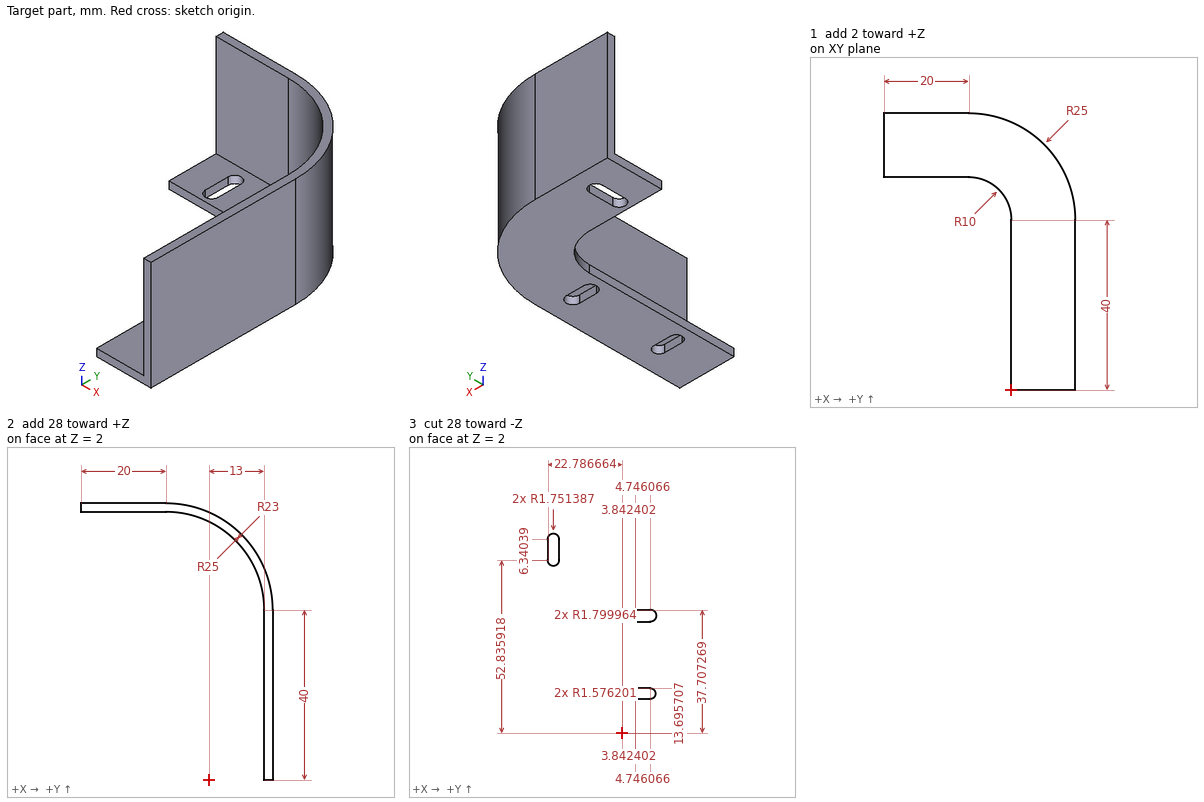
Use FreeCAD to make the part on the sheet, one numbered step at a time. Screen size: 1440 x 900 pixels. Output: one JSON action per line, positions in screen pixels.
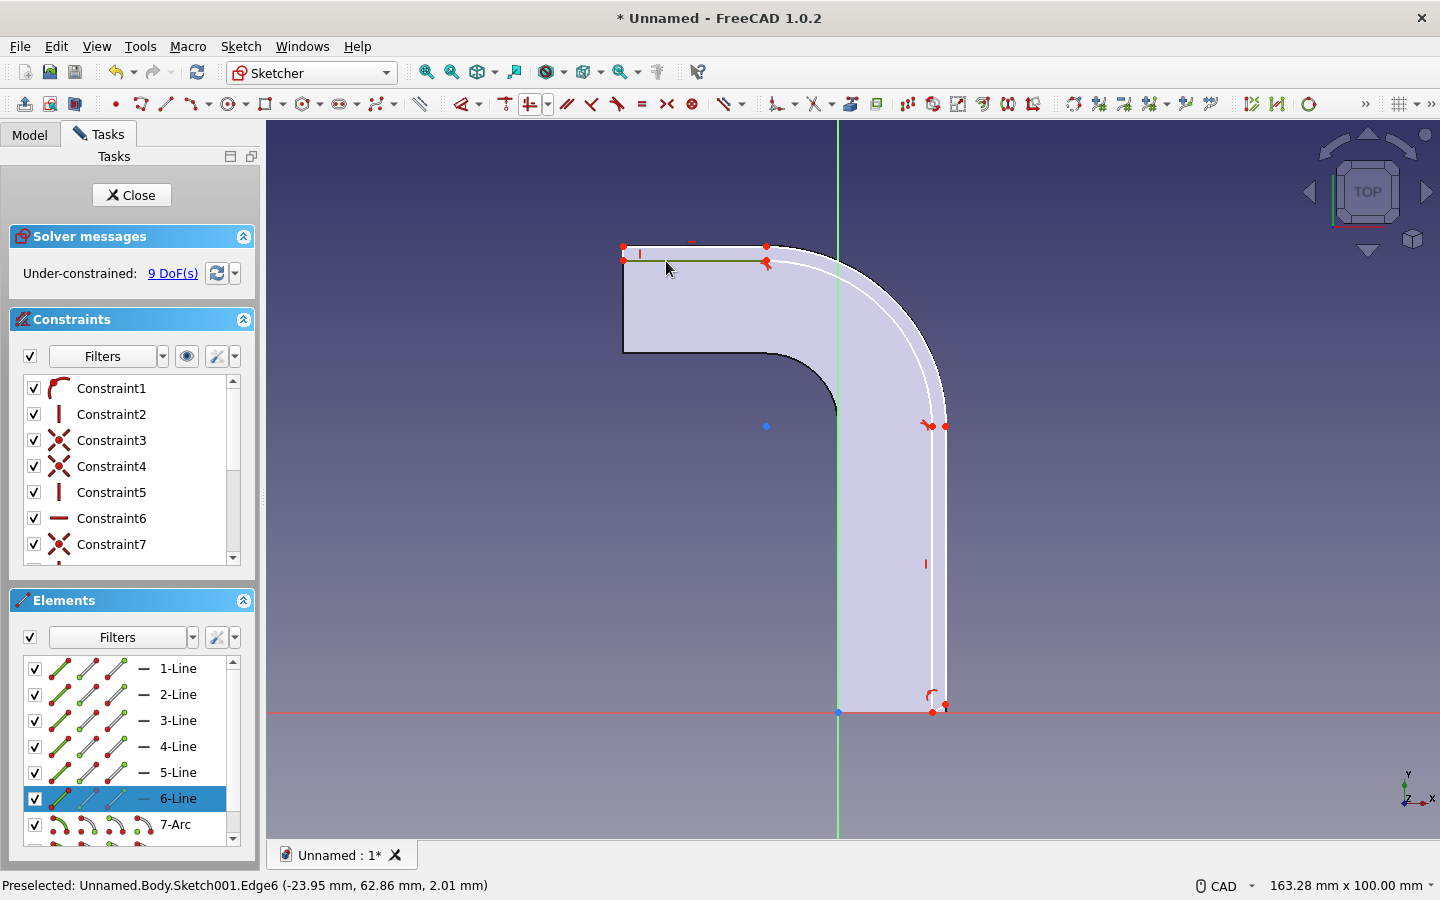
{"action": "left_click", "coordinate": [914, 351]}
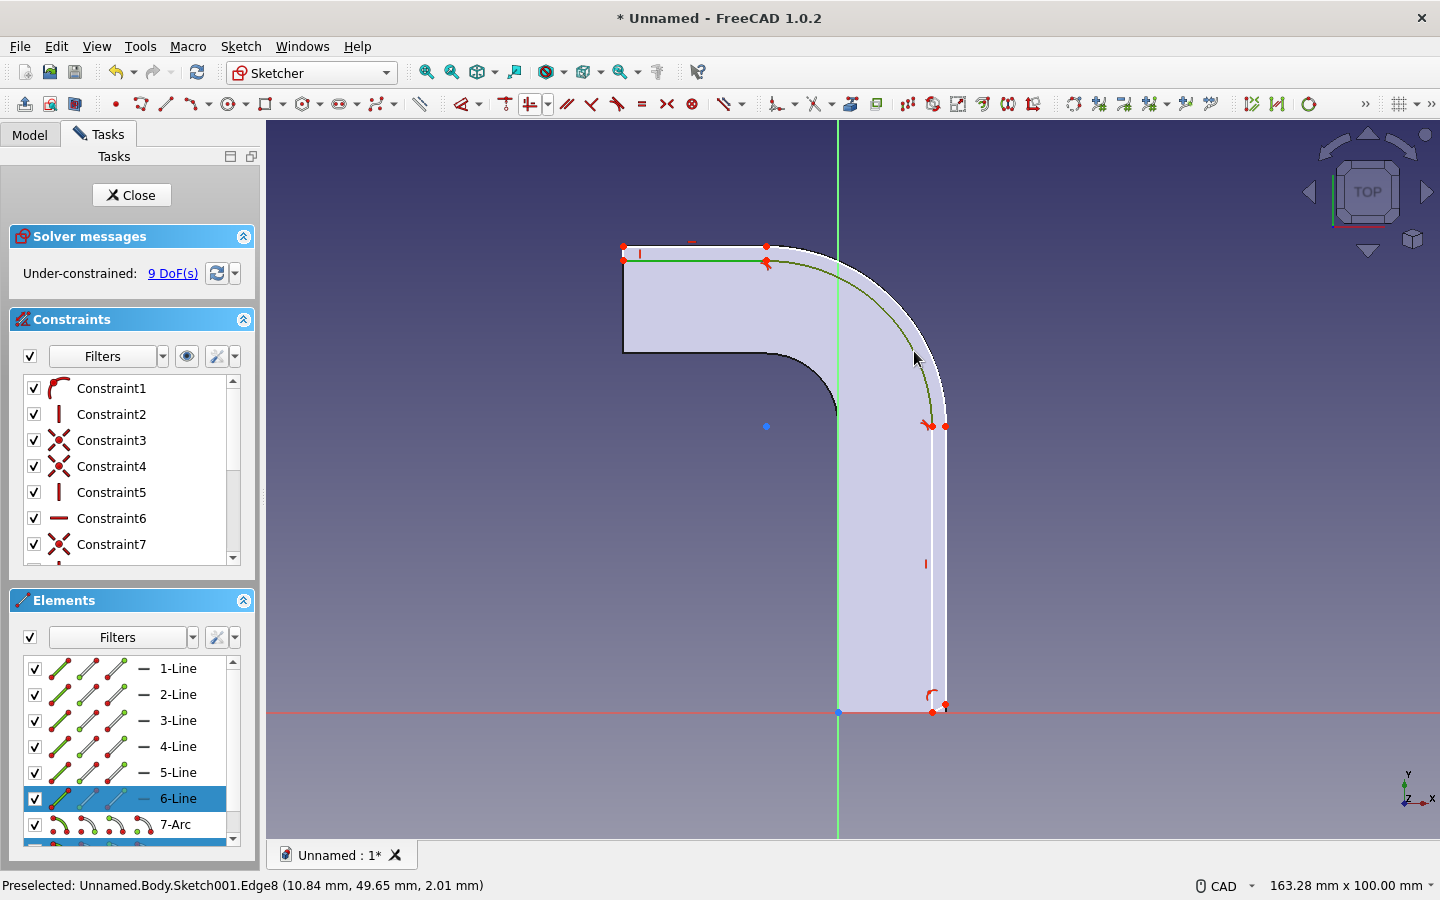
{"action": "key", "text": "t"}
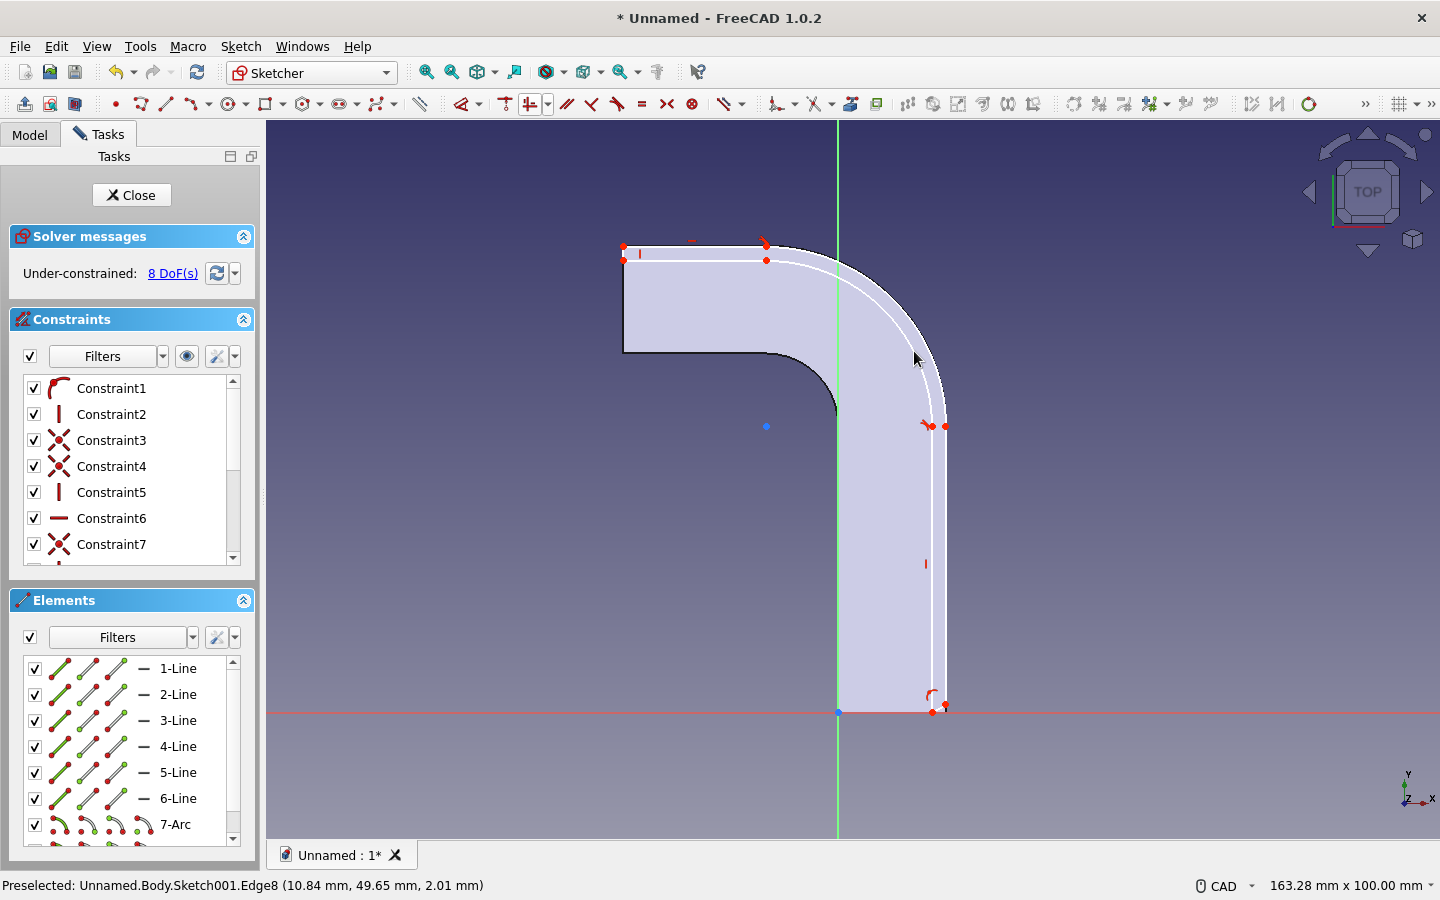
{"action": "scroll", "coordinate": [939, 709], "scroll_direction": "up", "scroll_amount": 4}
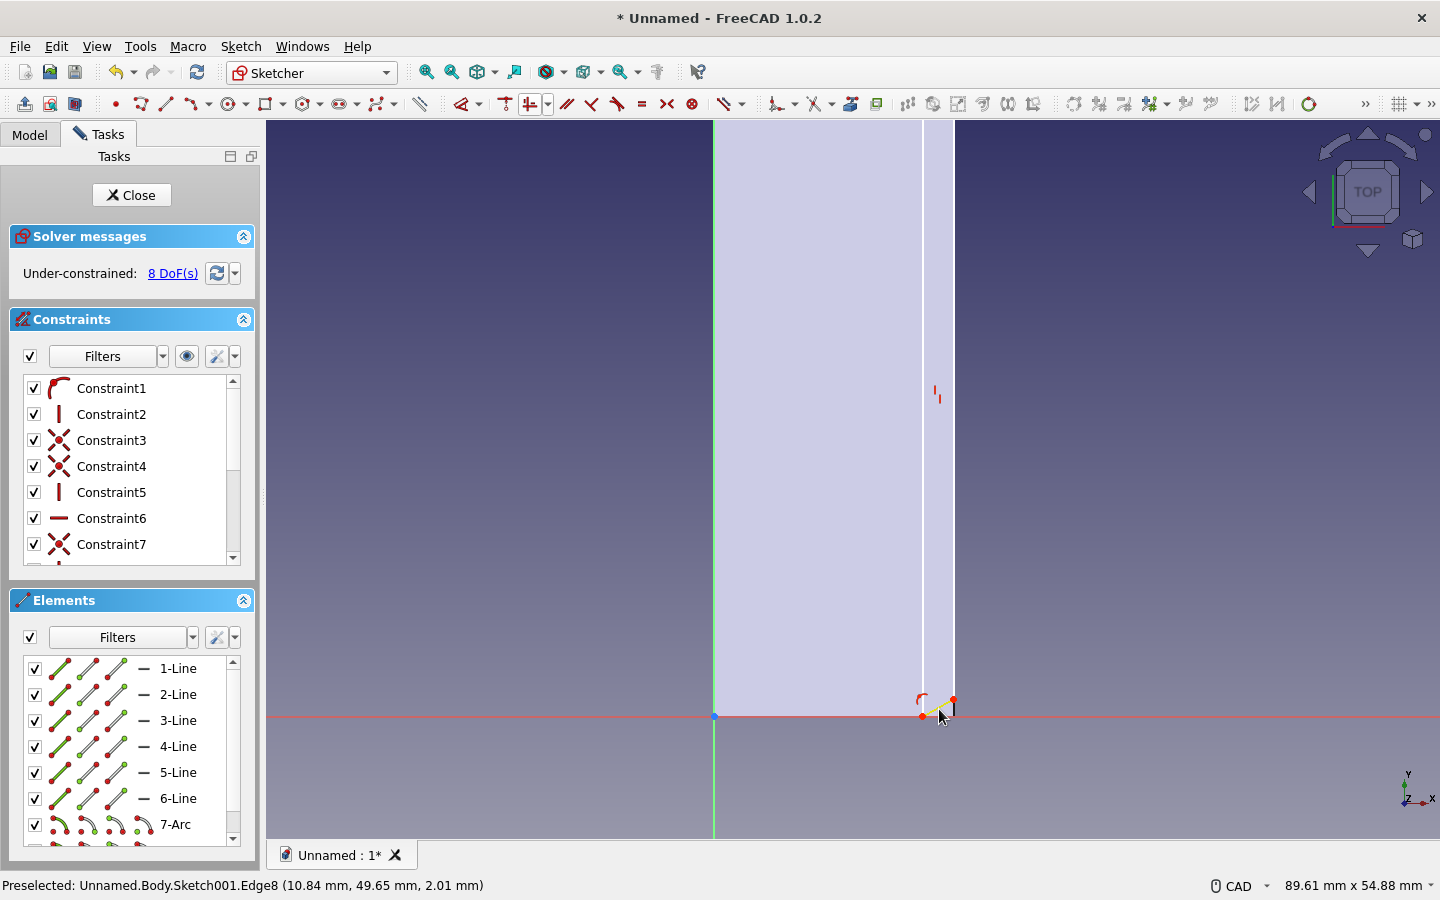
{"action": "left_click", "coordinate": [938, 708]}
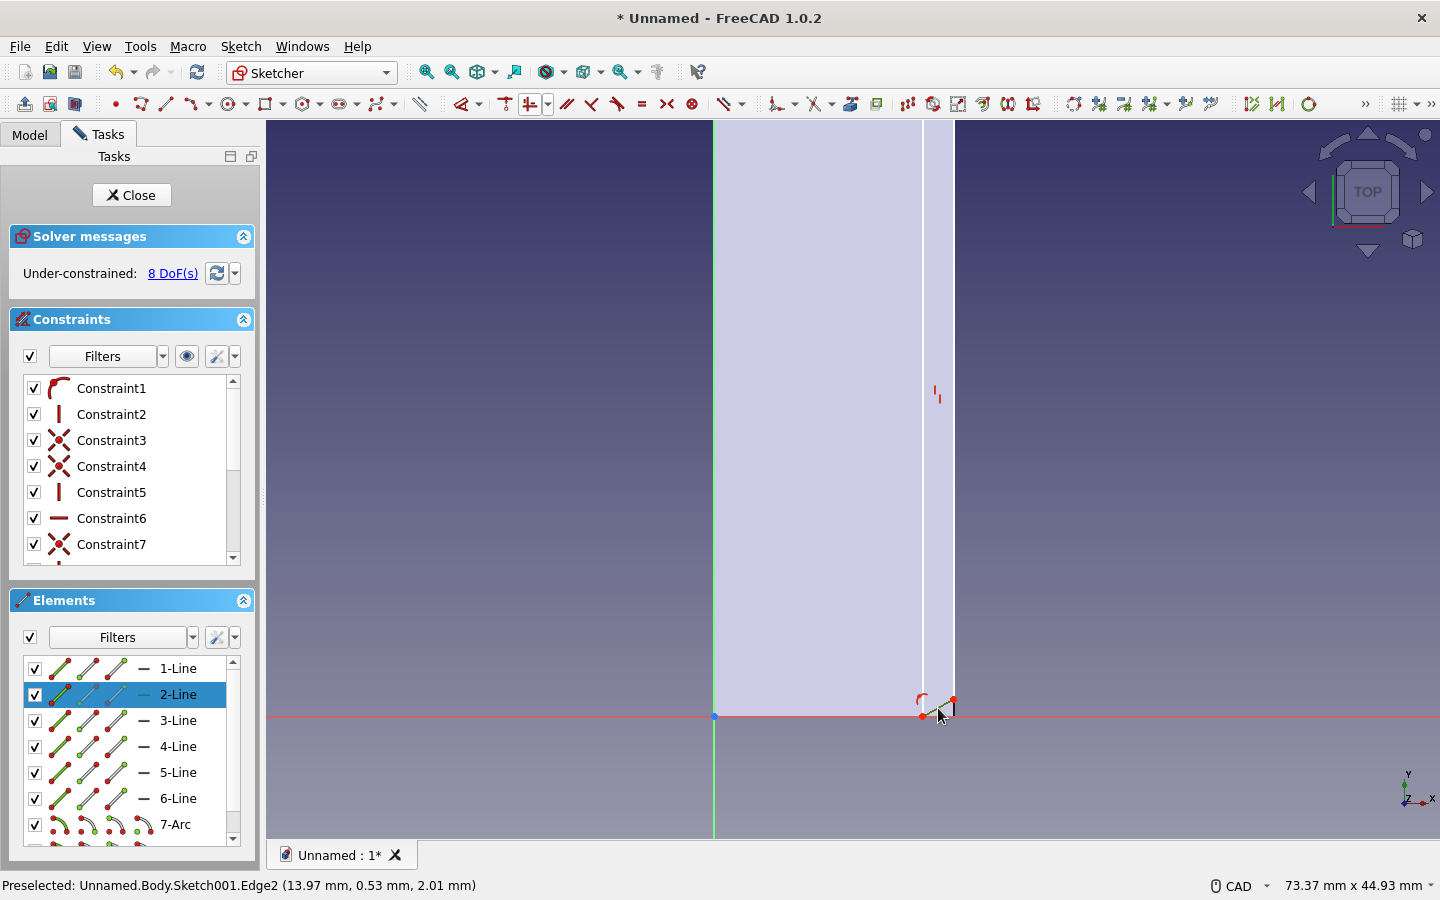
{"action": "left_click", "coordinate": [548, 104]}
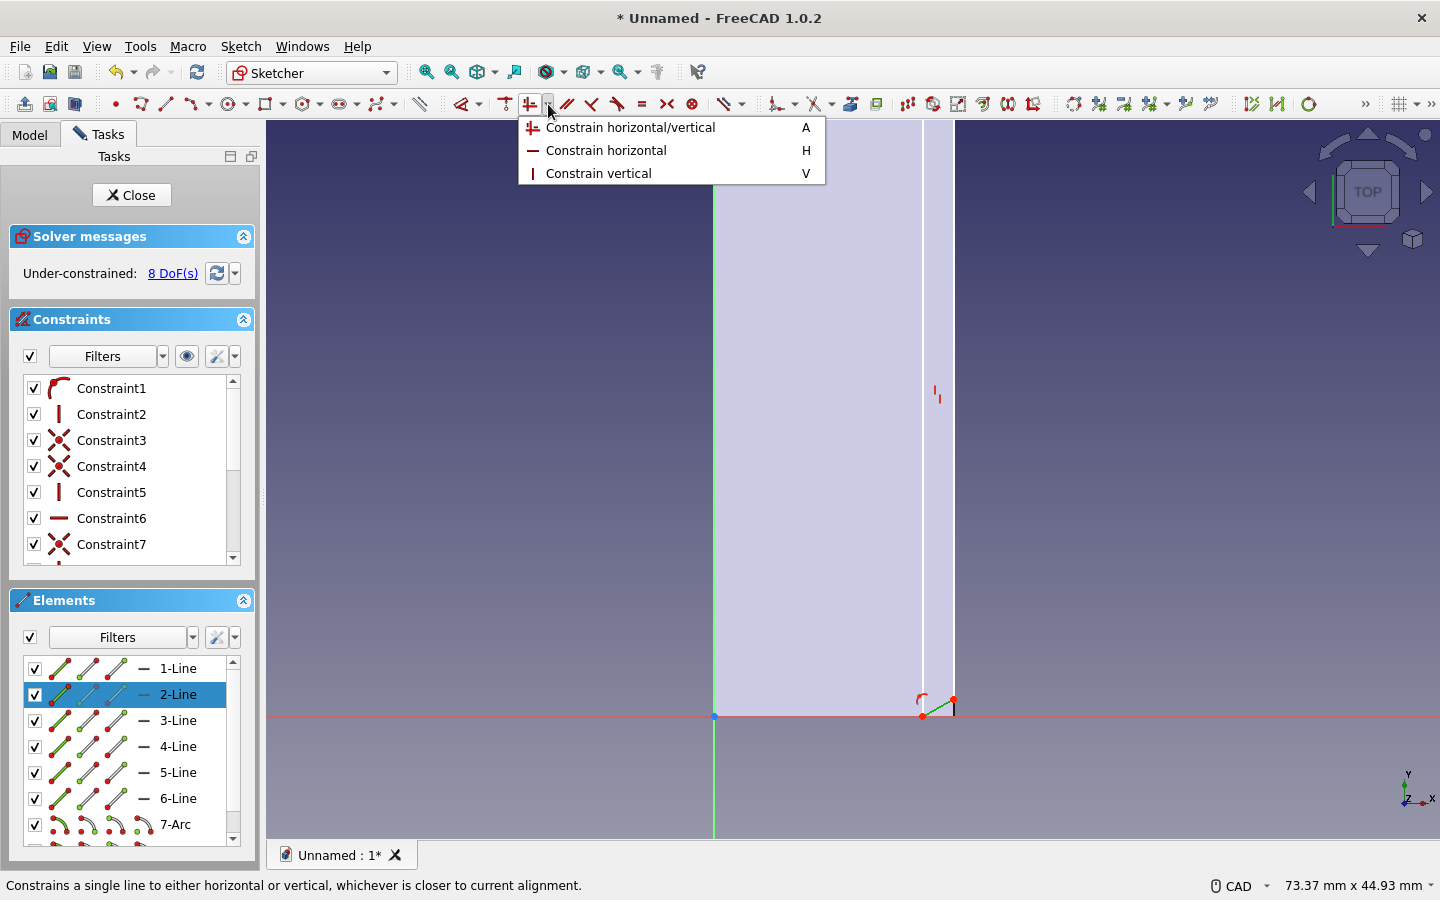
{"action": "left_click", "coordinate": [672, 150]}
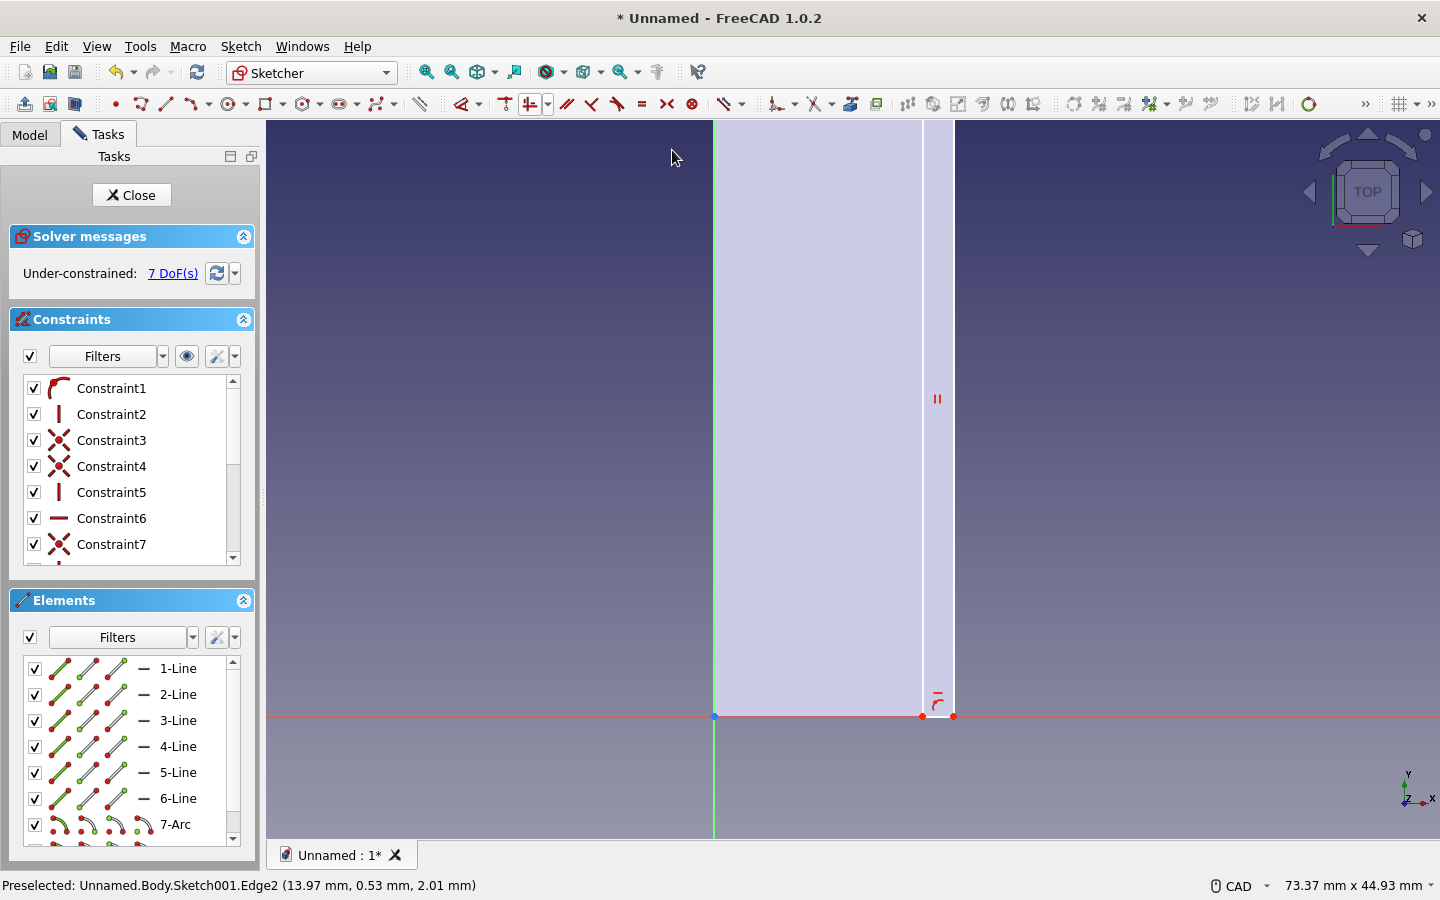
{"action": "scroll", "coordinate": [940, 710], "scroll_direction": "down", "scroll_amount": 4}